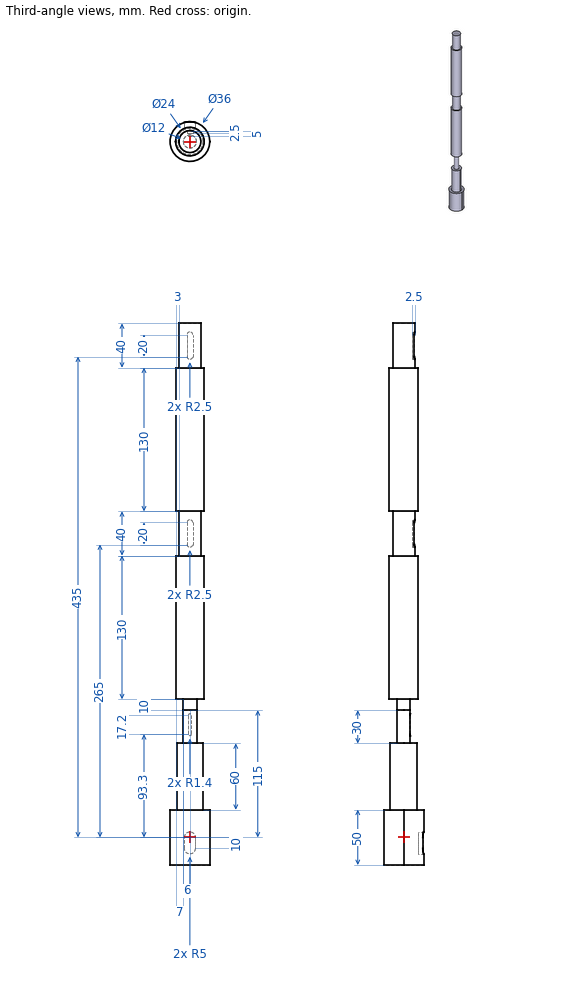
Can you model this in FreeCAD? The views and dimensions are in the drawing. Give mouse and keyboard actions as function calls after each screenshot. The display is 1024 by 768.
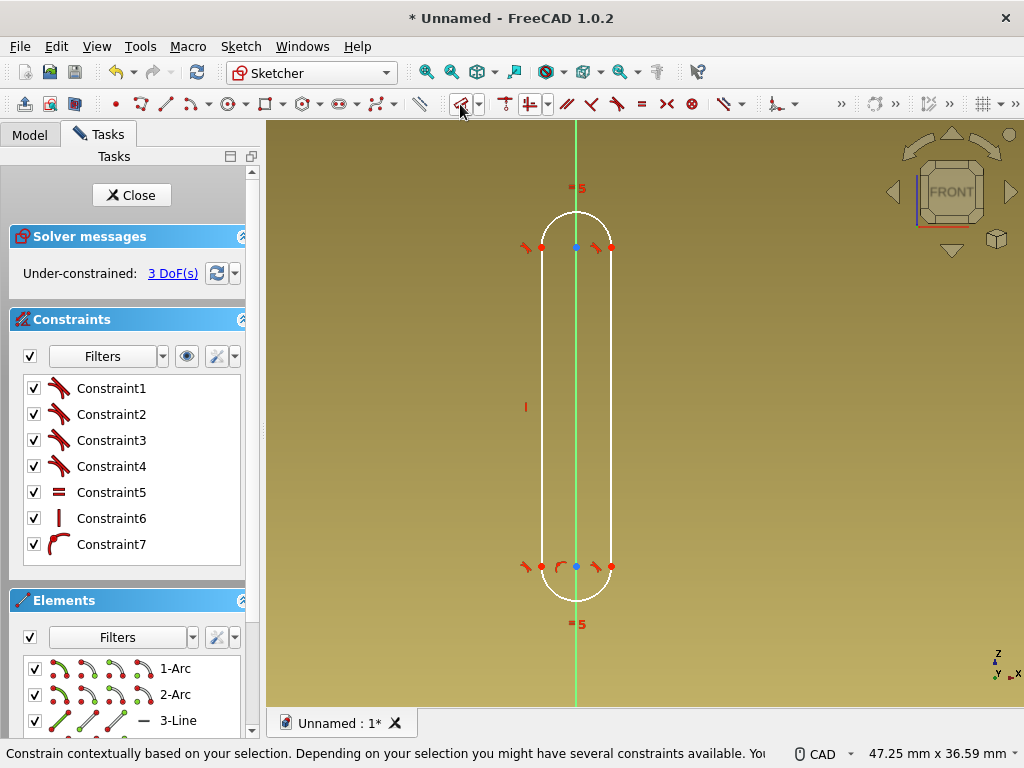
click(556, 594)
click(537, 620)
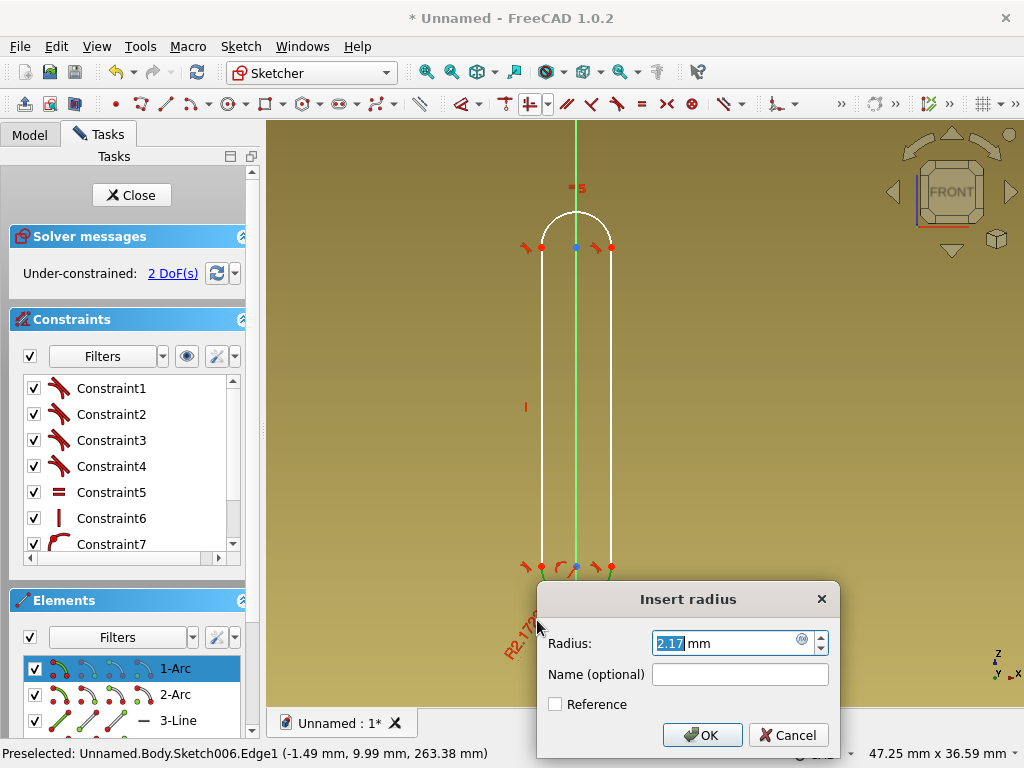
text(2.5)
key(Return)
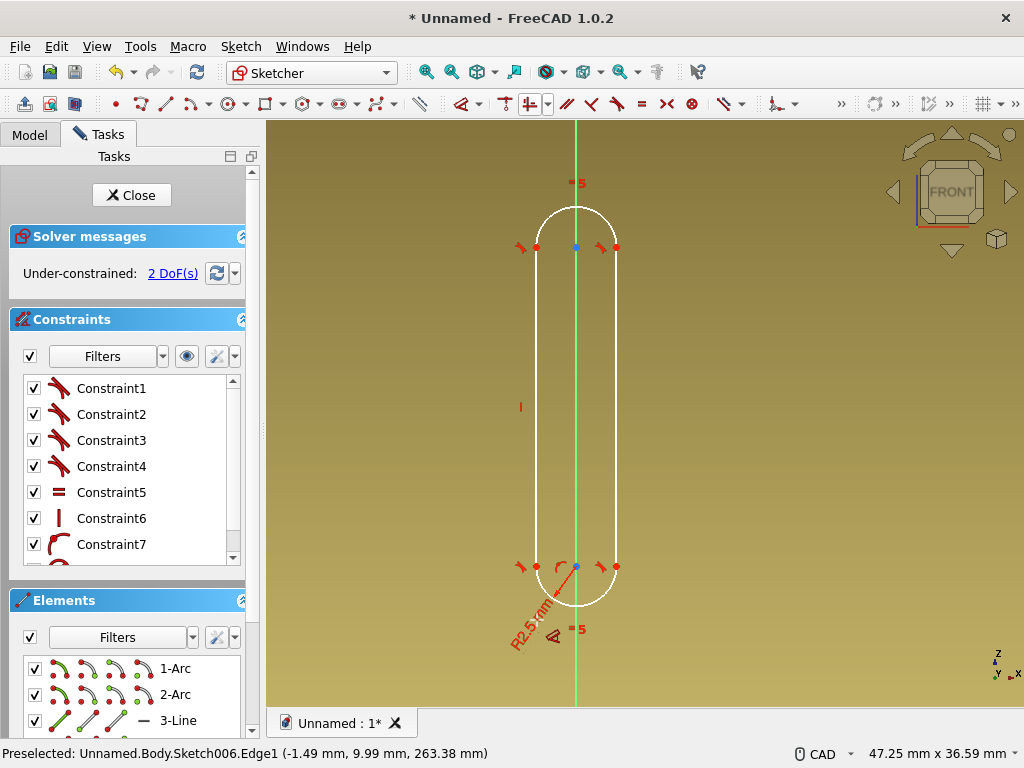
click(536, 470)
click(502, 407)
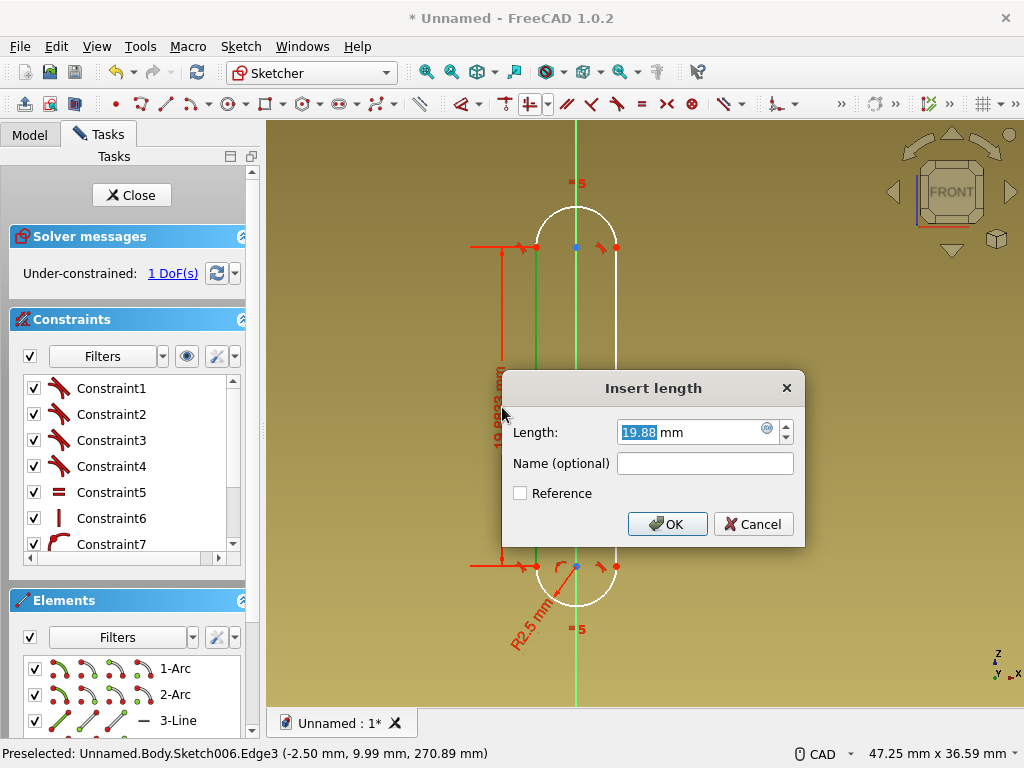
text(20)
key(Return)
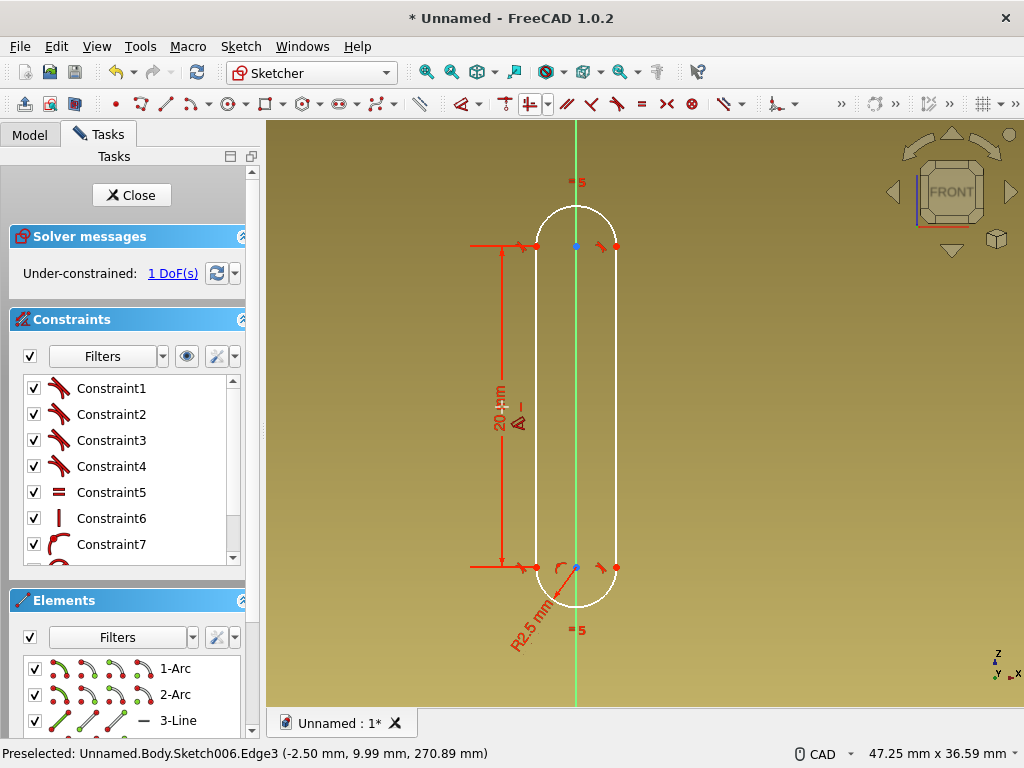
click(536, 567)
click(502, 597)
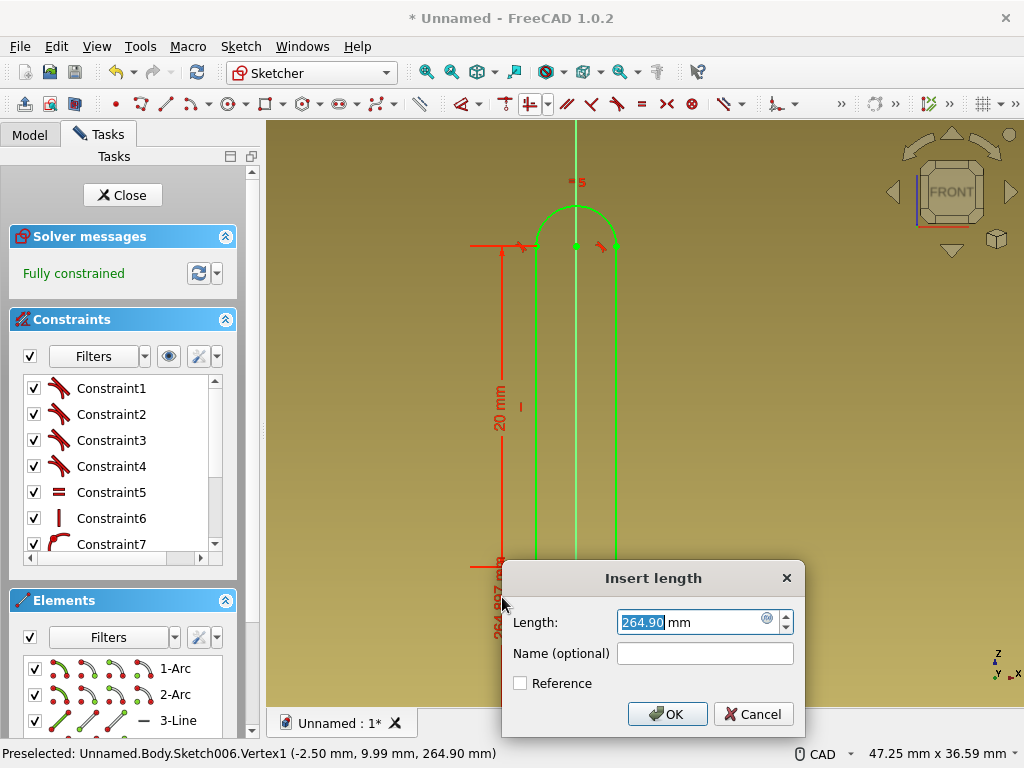
text(265)
key(Return)
key(Escape)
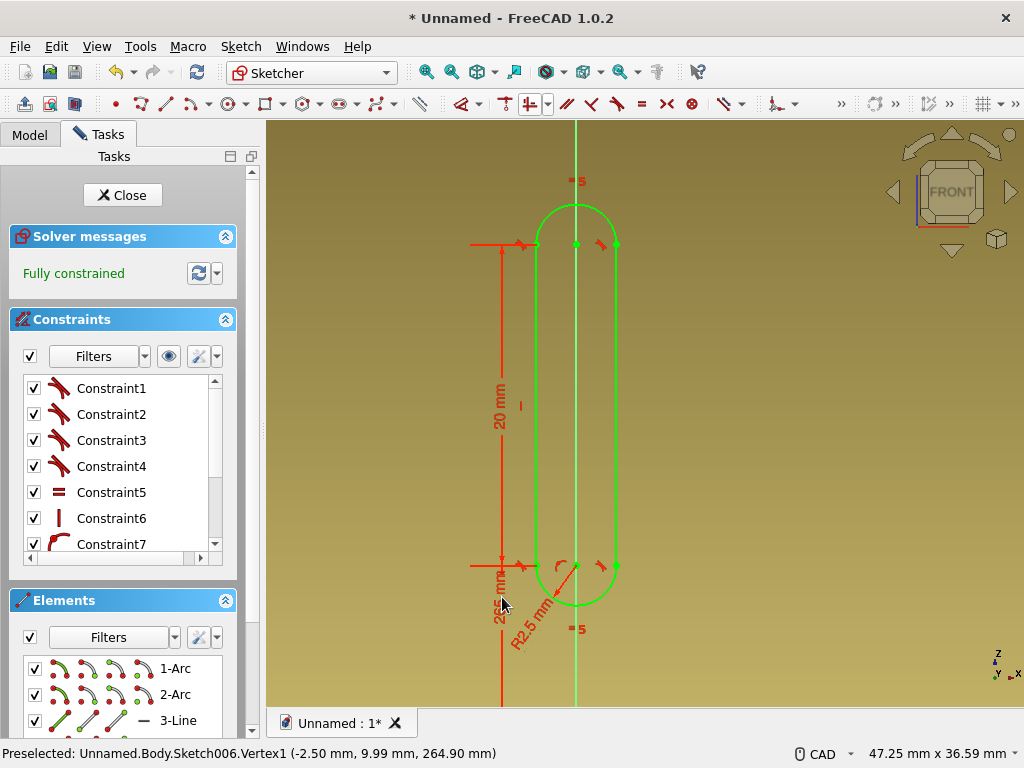
click(123, 195)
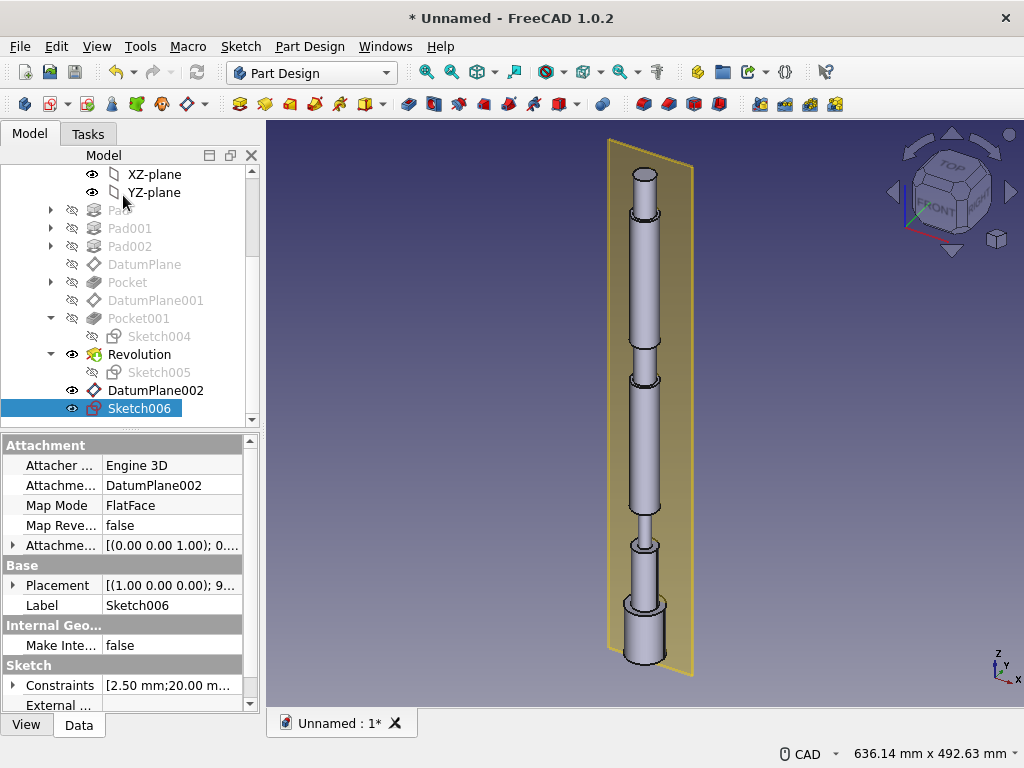
click(409, 104)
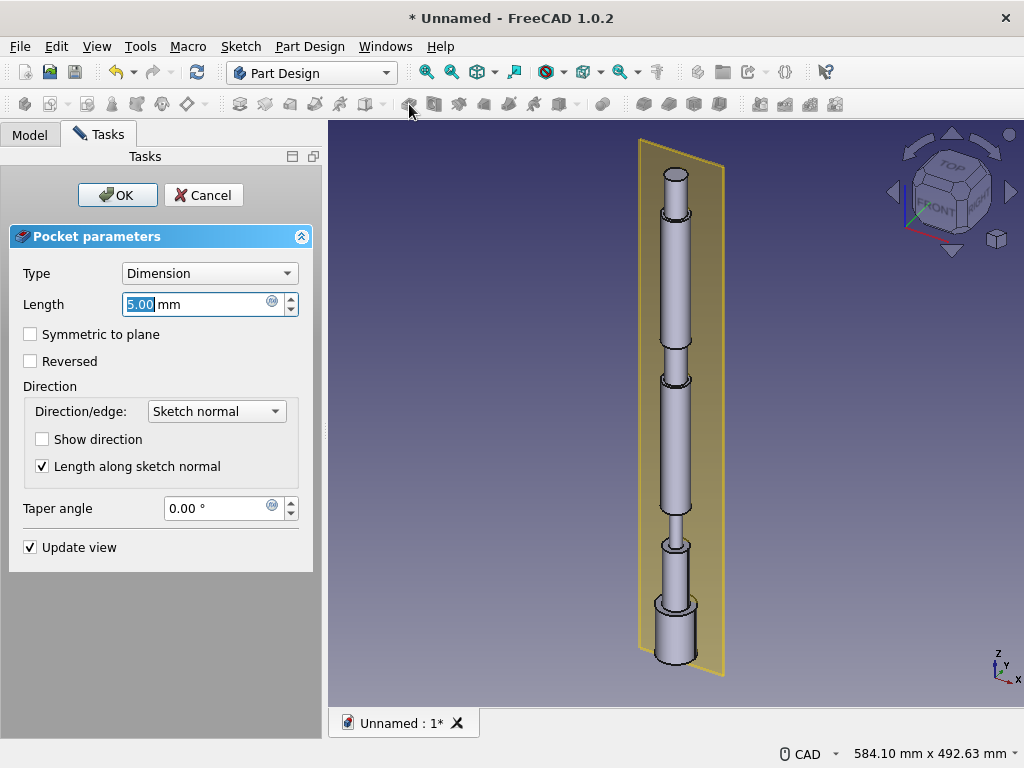
text(2.5)
key(Tab)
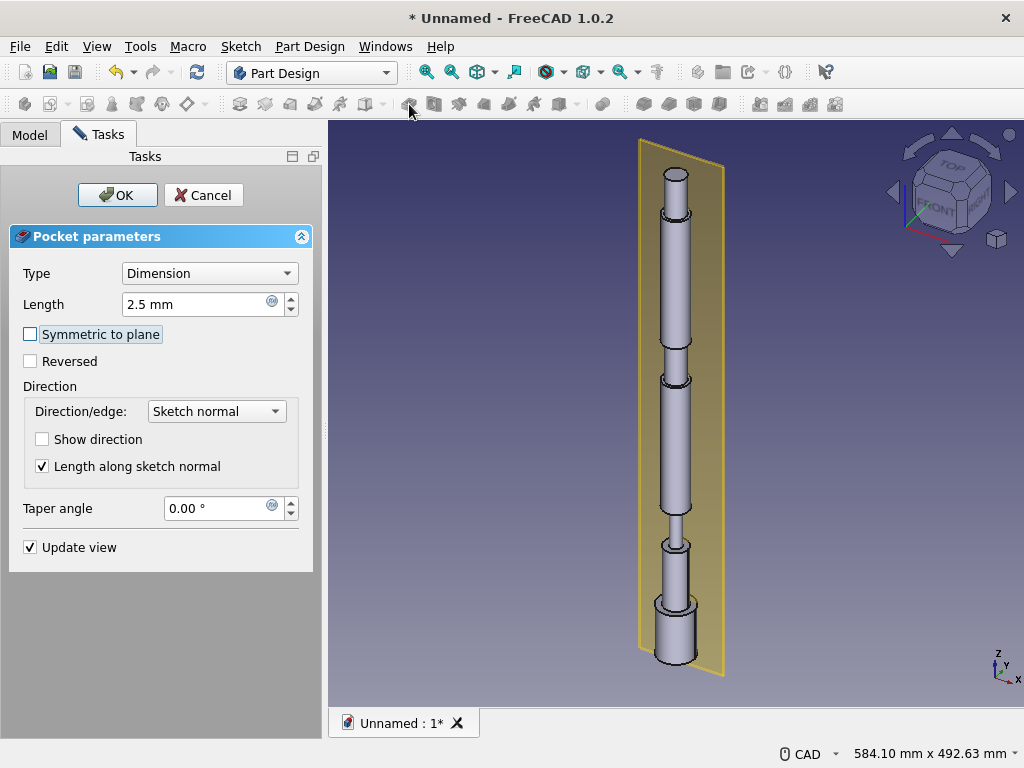
click(31, 361)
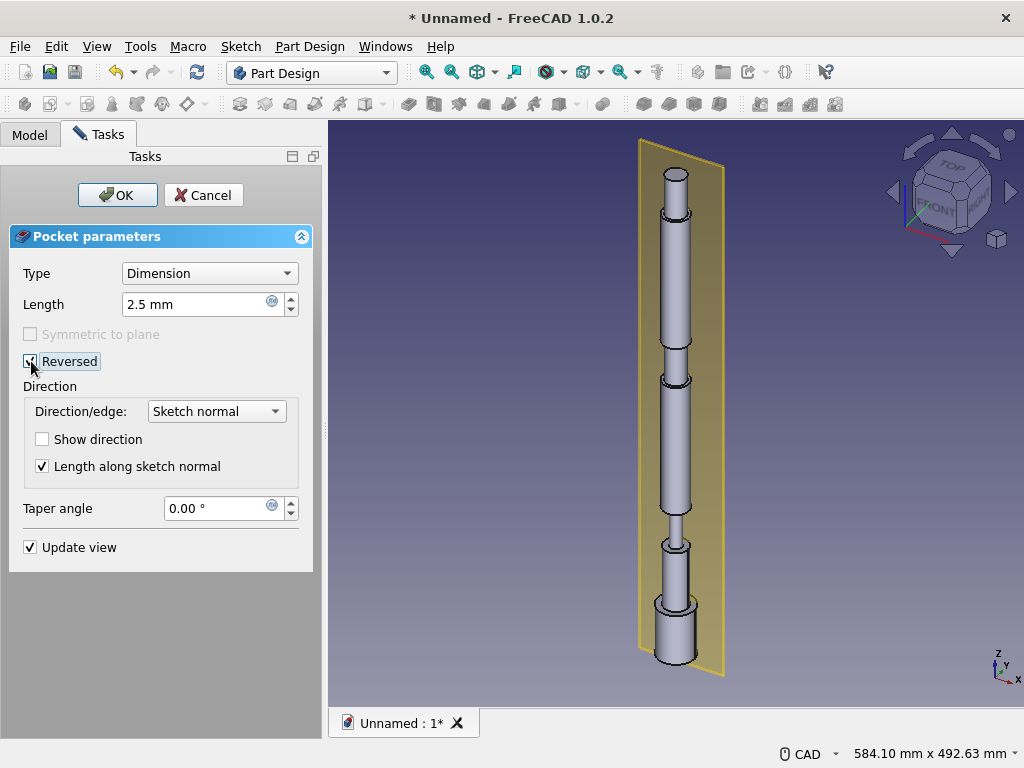
click(118, 195)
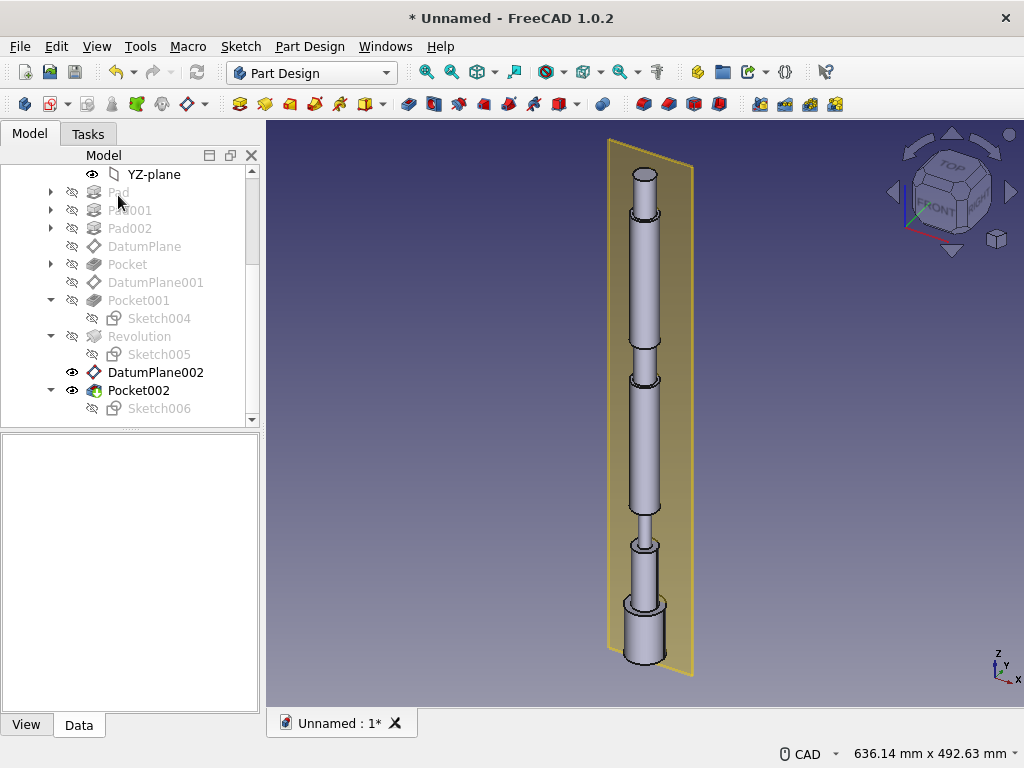
click(117, 372)
key(space)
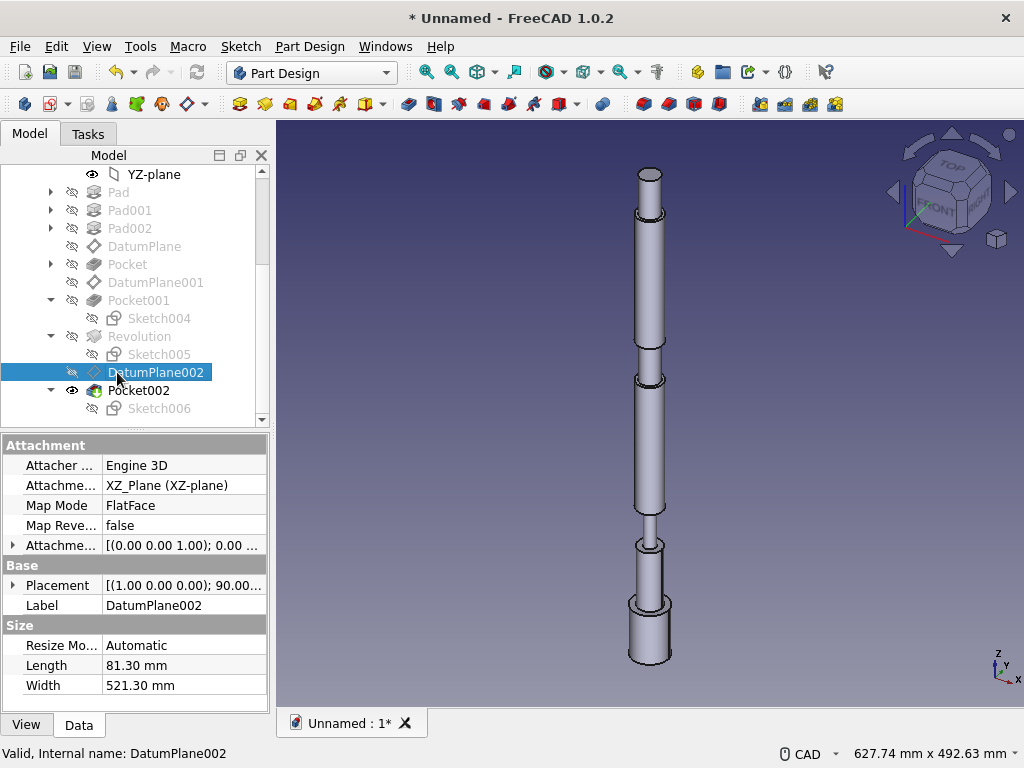
scroll(161, 296, down, 3)